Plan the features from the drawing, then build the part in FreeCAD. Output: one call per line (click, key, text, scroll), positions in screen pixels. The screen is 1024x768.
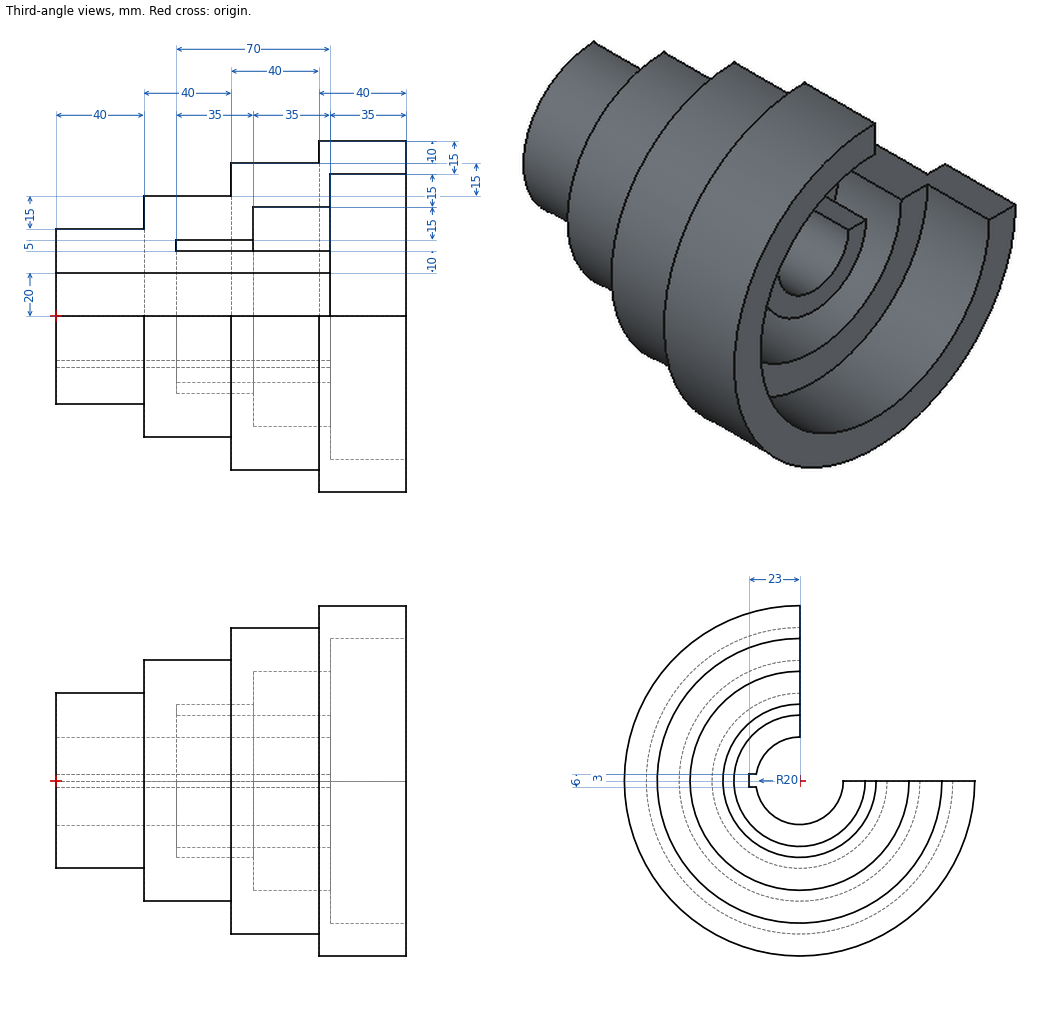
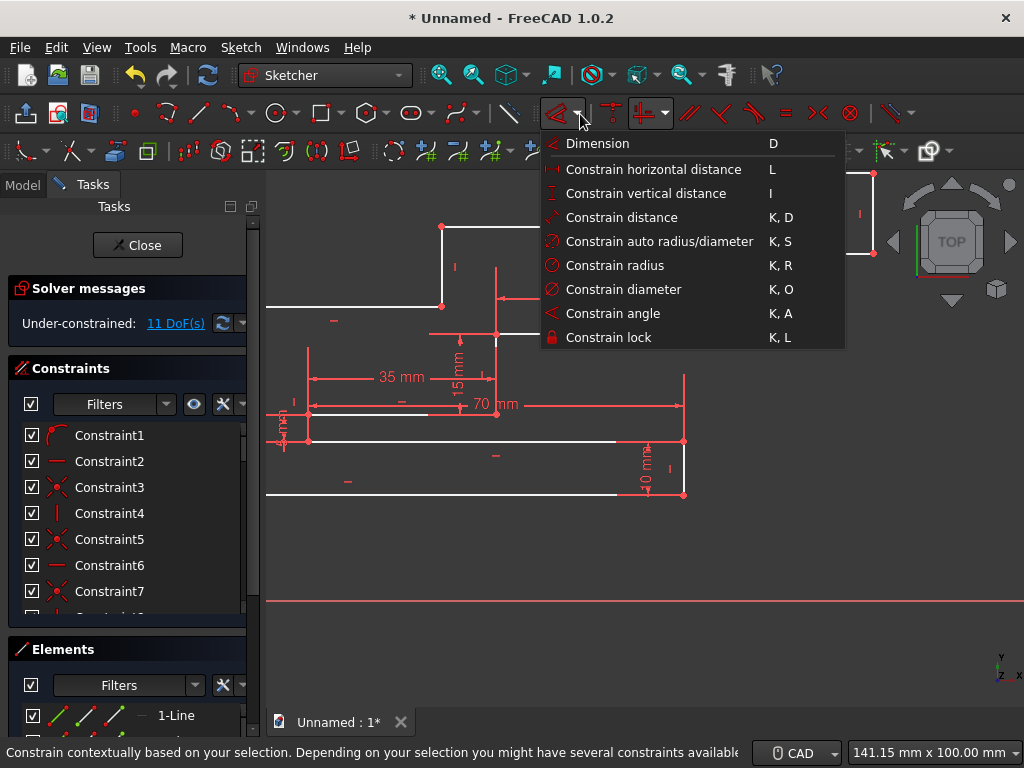
click(693, 193)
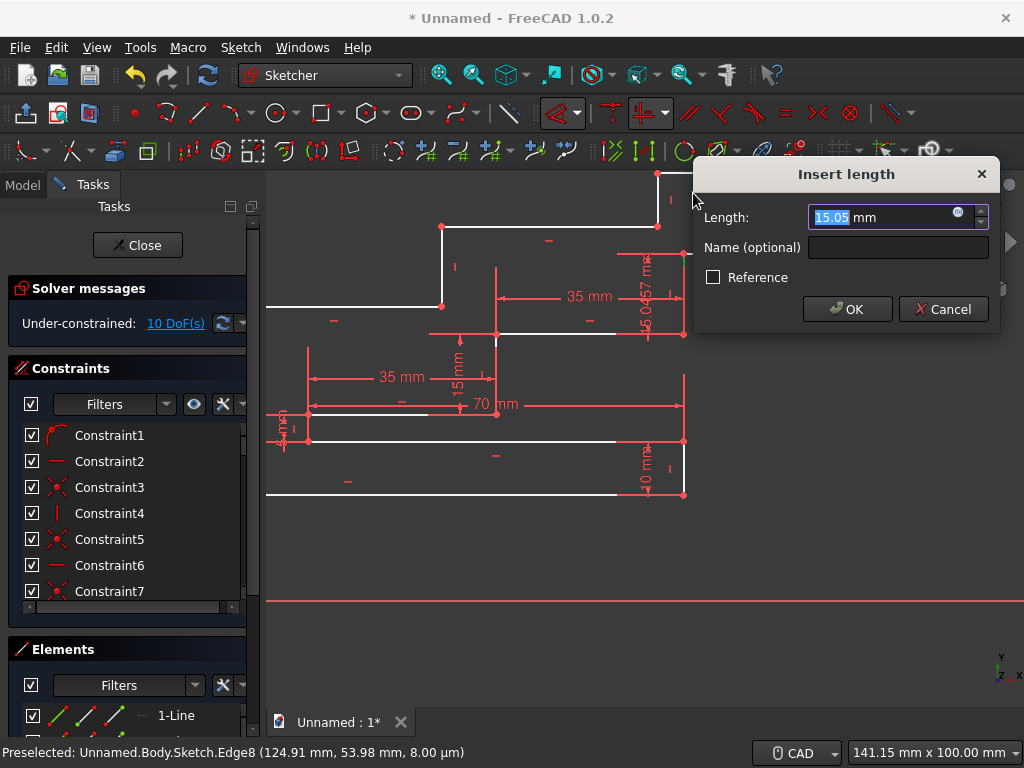
text(15)
key(Return)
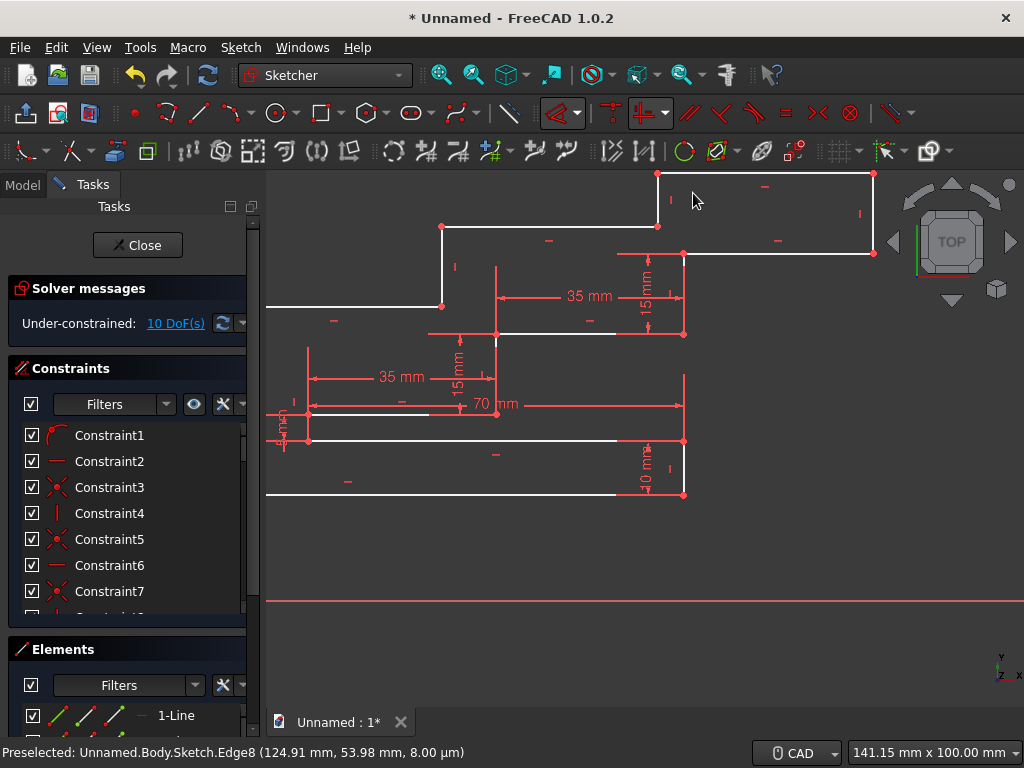
click(741, 254)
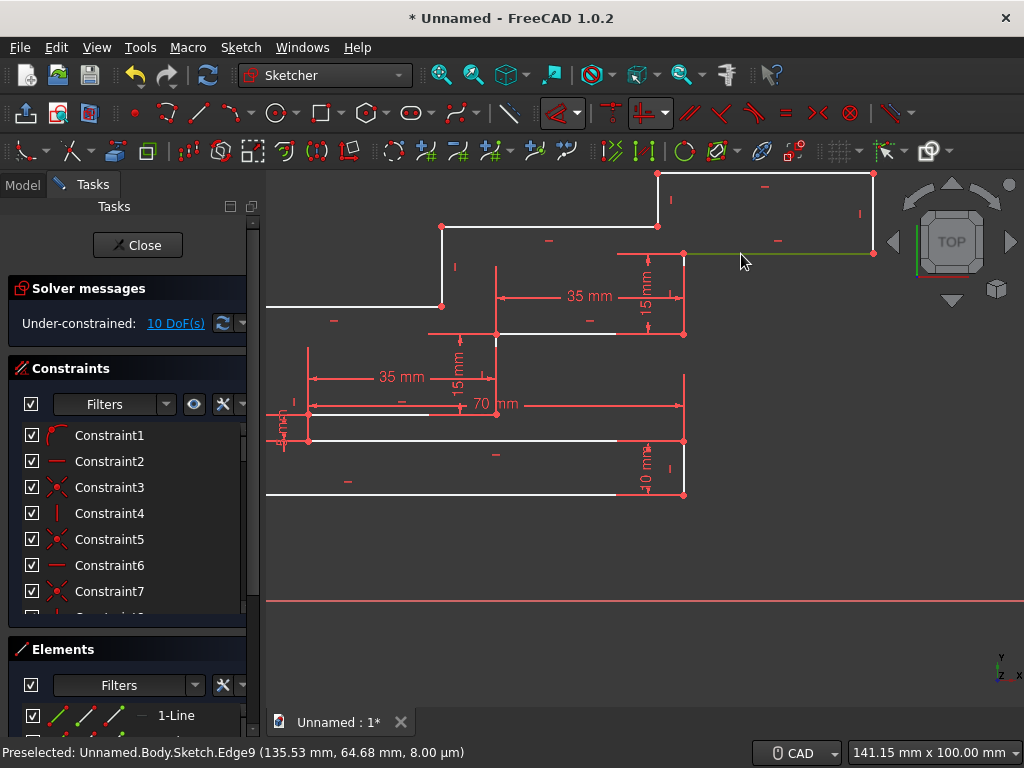
key(l)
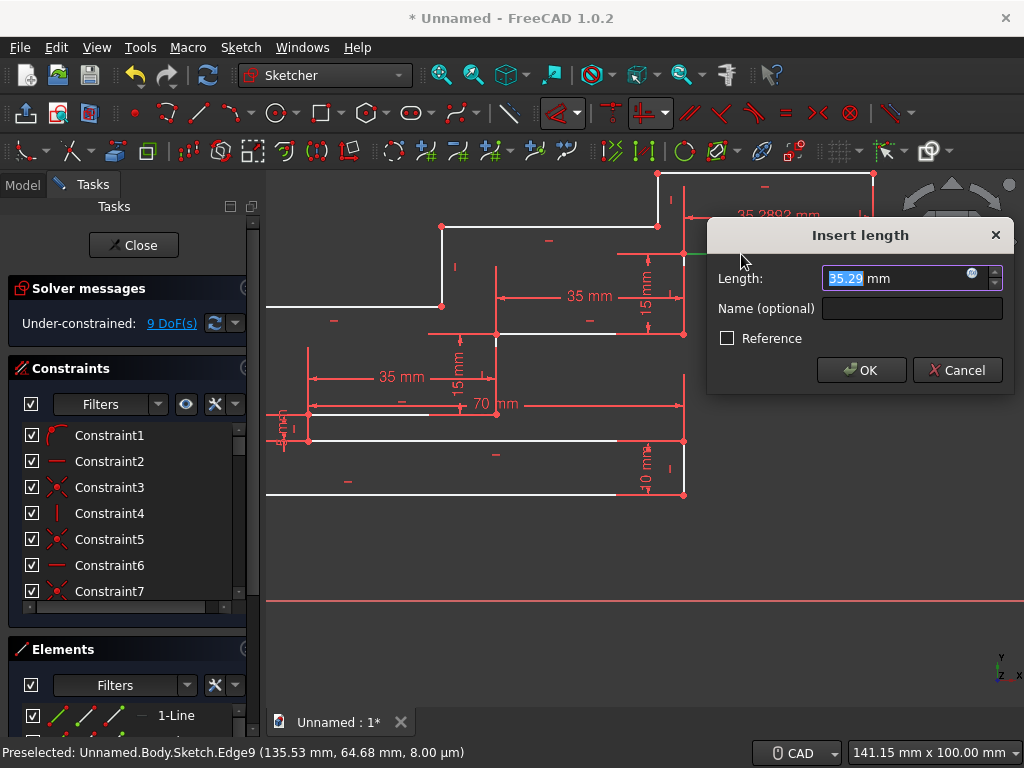
text(35)
key(Return)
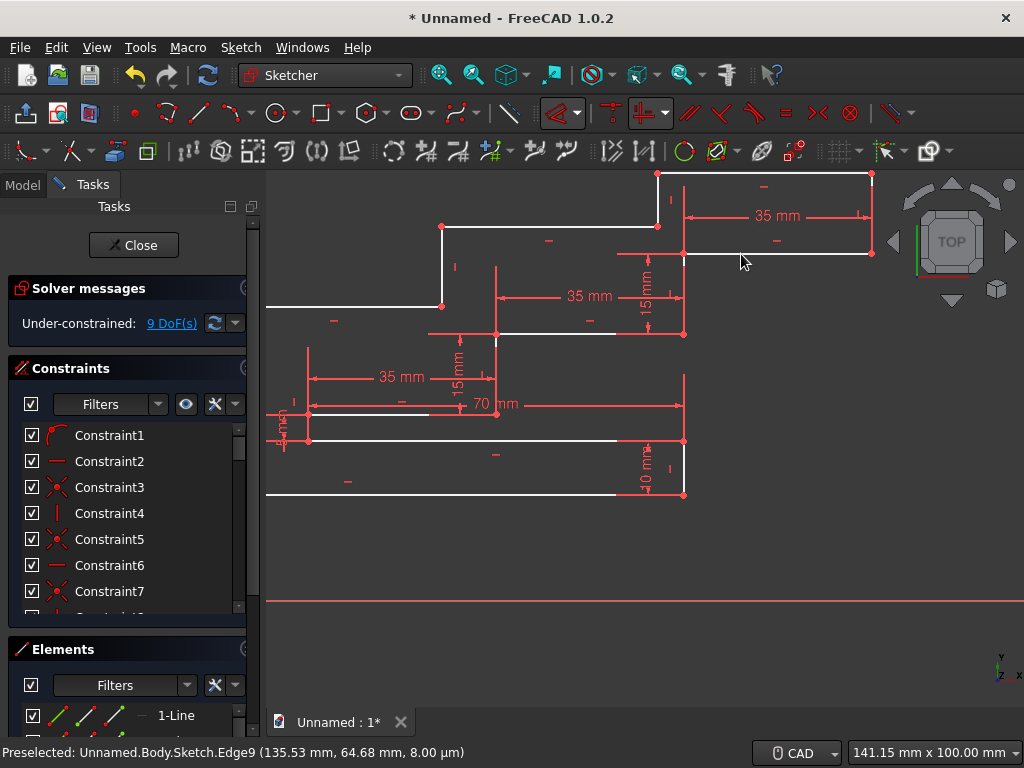
scroll(686, 481, down, 4)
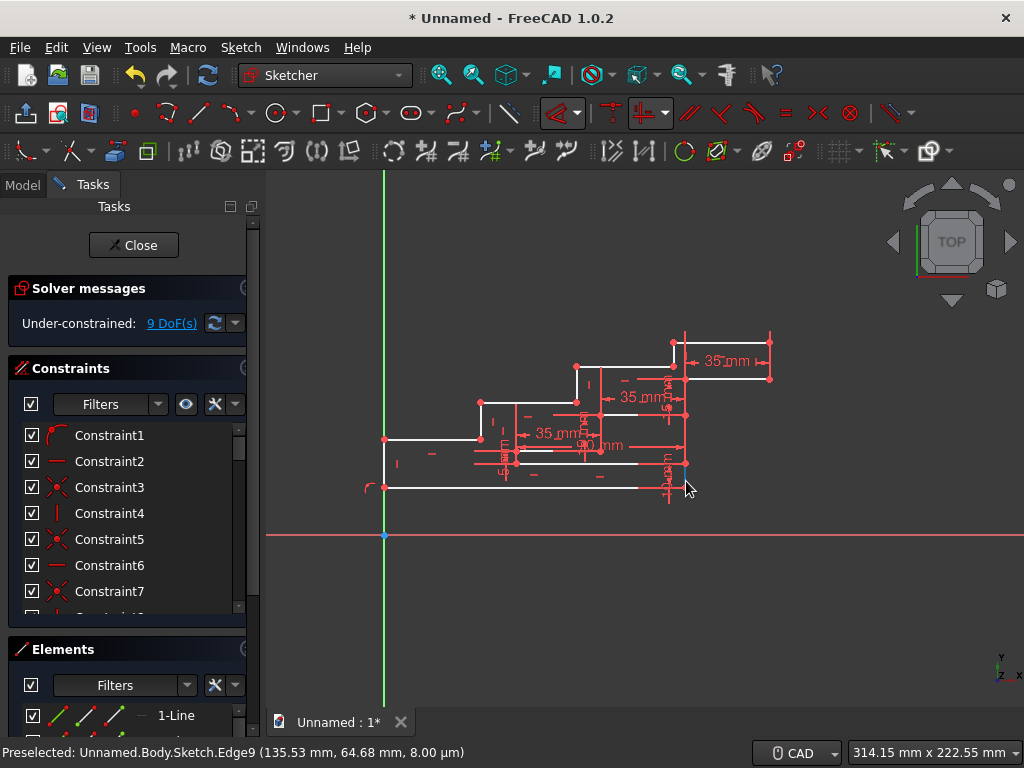
scroll(770, 368, up, 2)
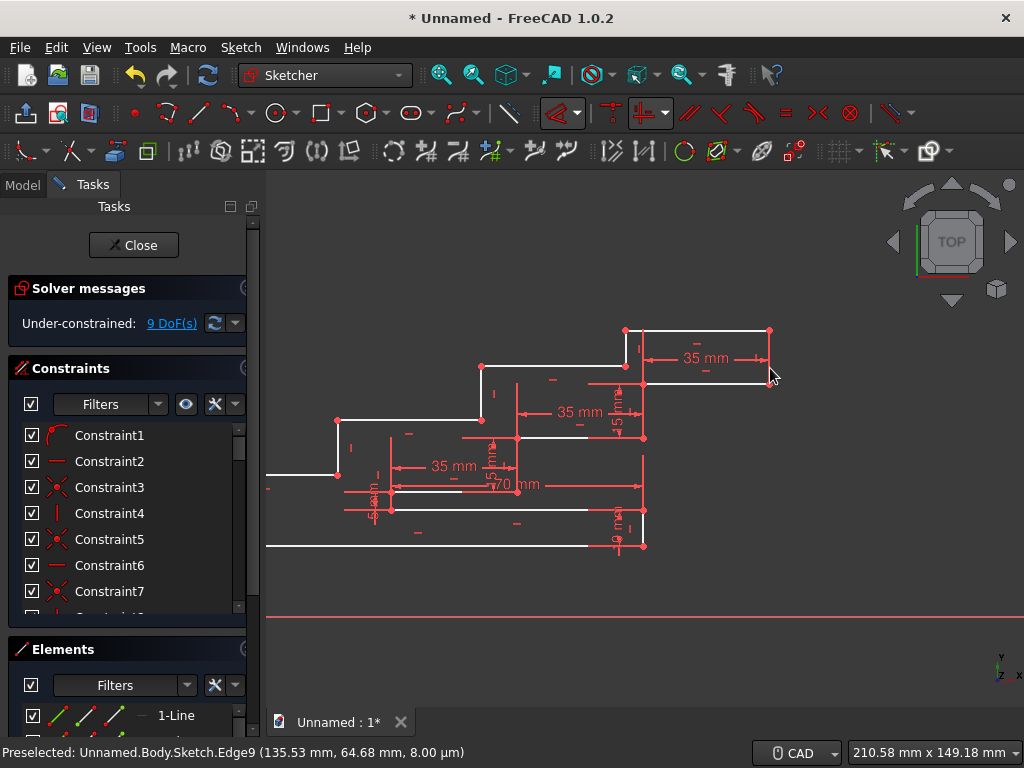
click(769, 368)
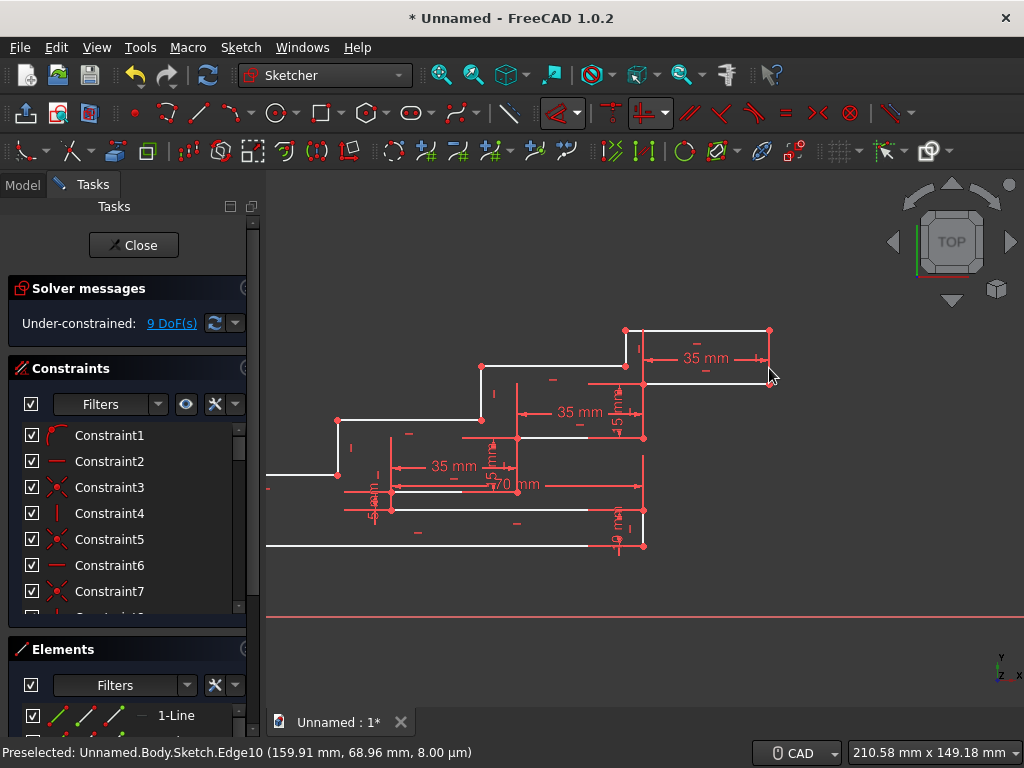
key(i)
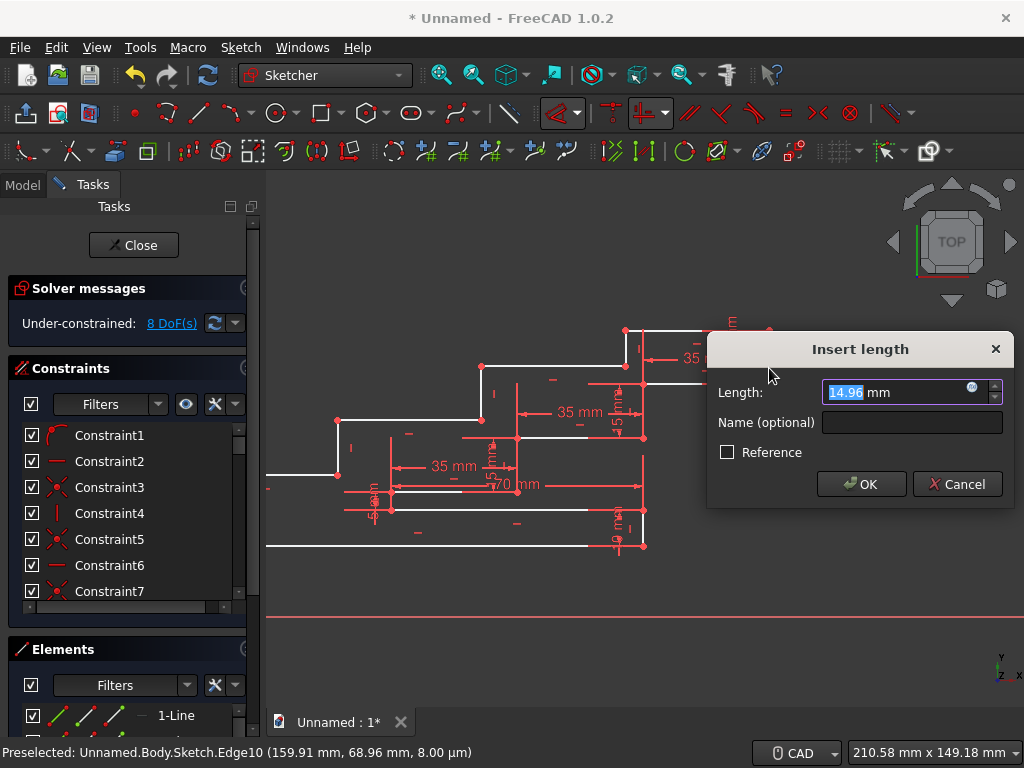
text(15)
key(Return)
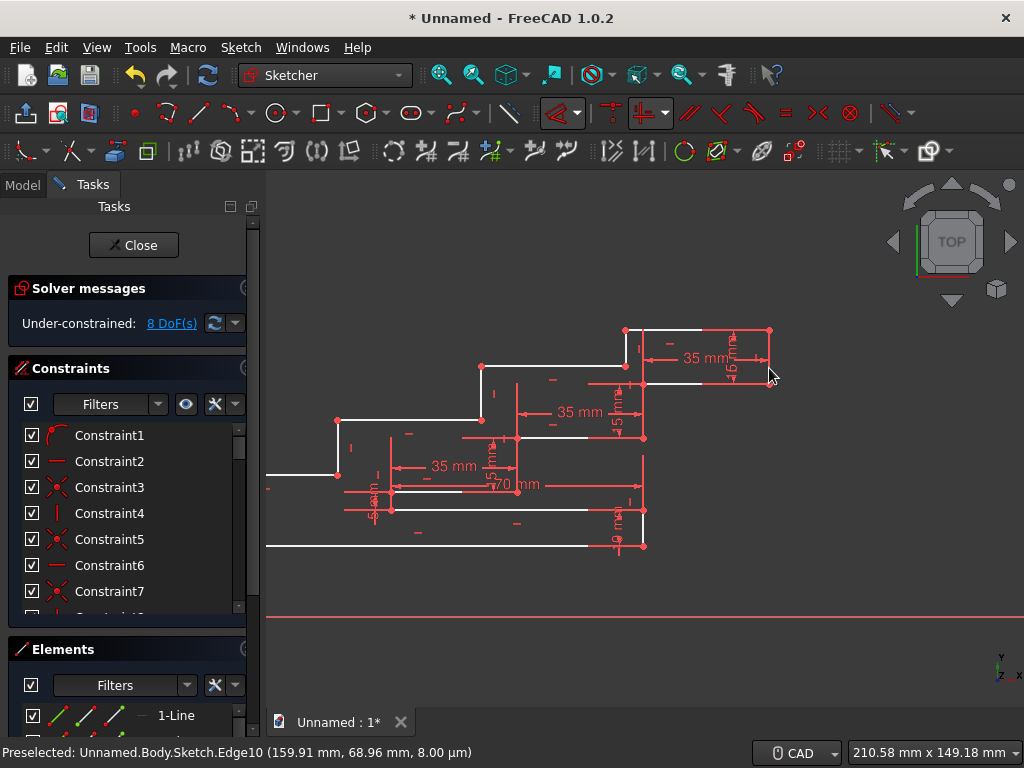
click(726, 330)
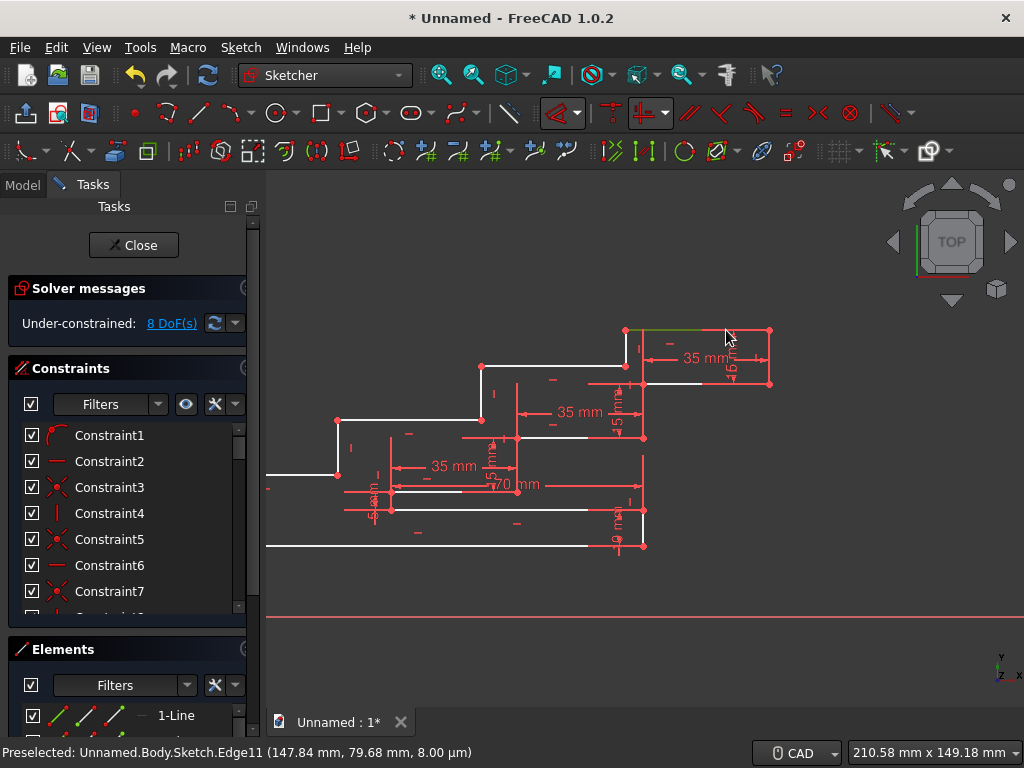
click(580, 114)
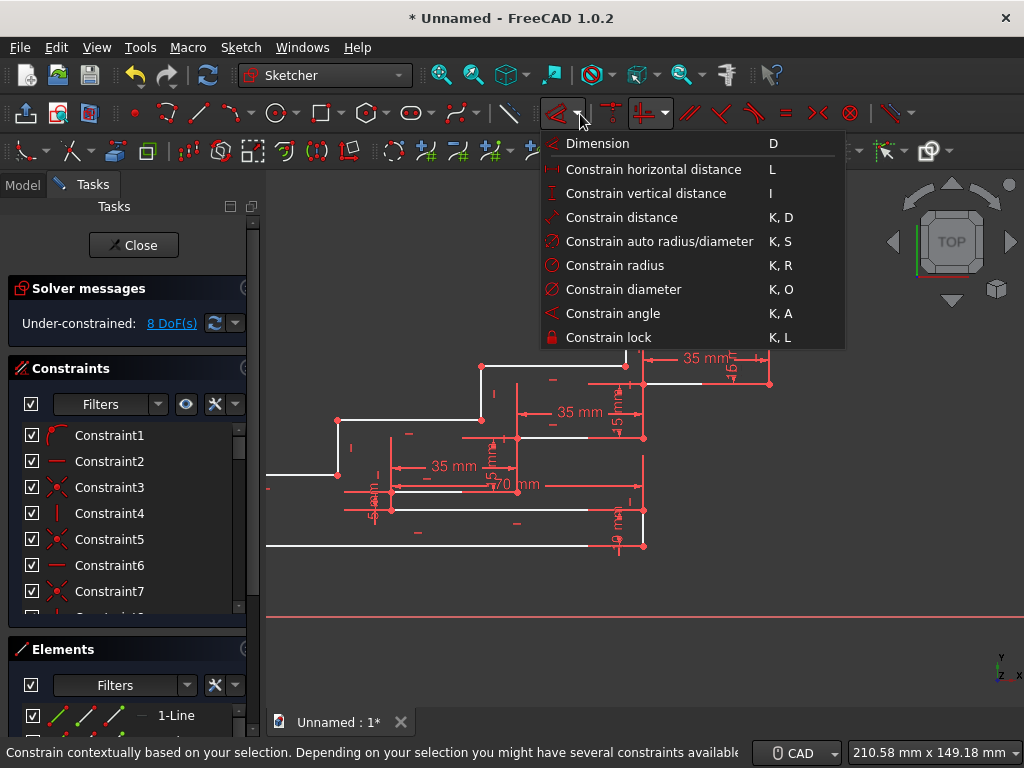
click(693, 169)